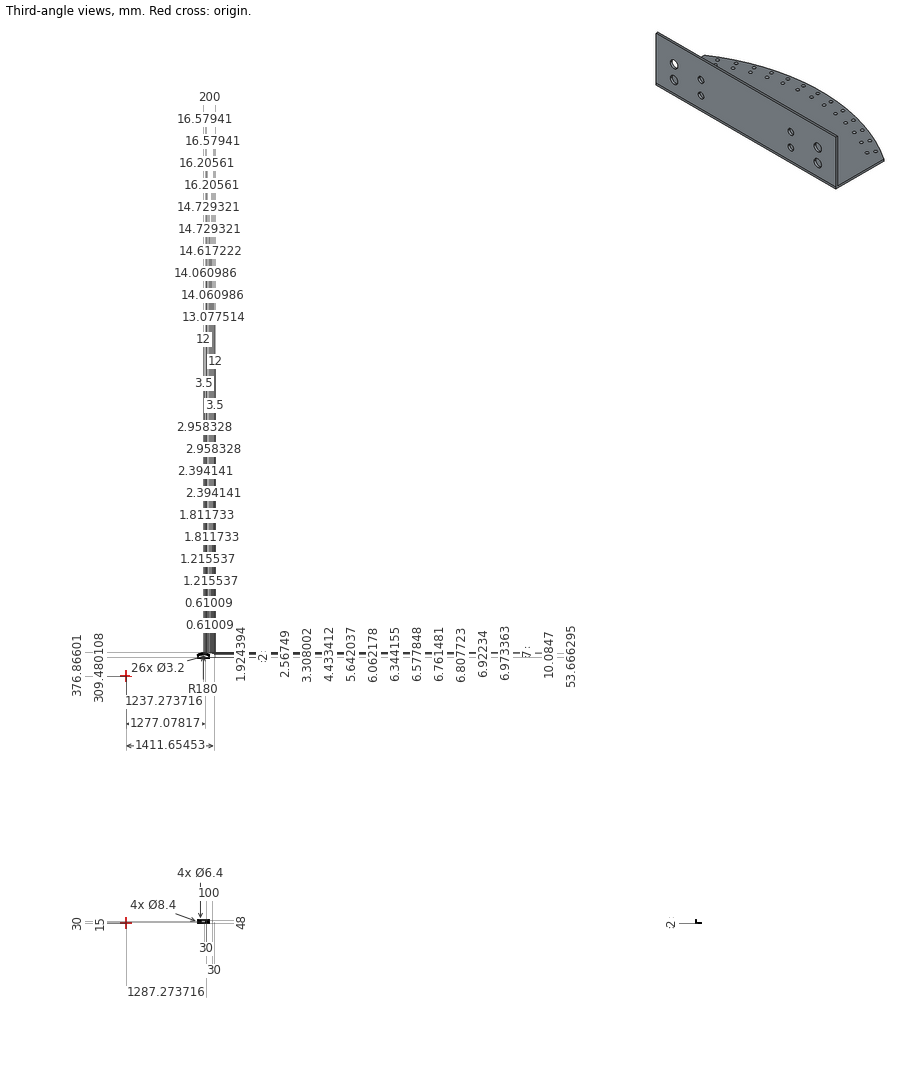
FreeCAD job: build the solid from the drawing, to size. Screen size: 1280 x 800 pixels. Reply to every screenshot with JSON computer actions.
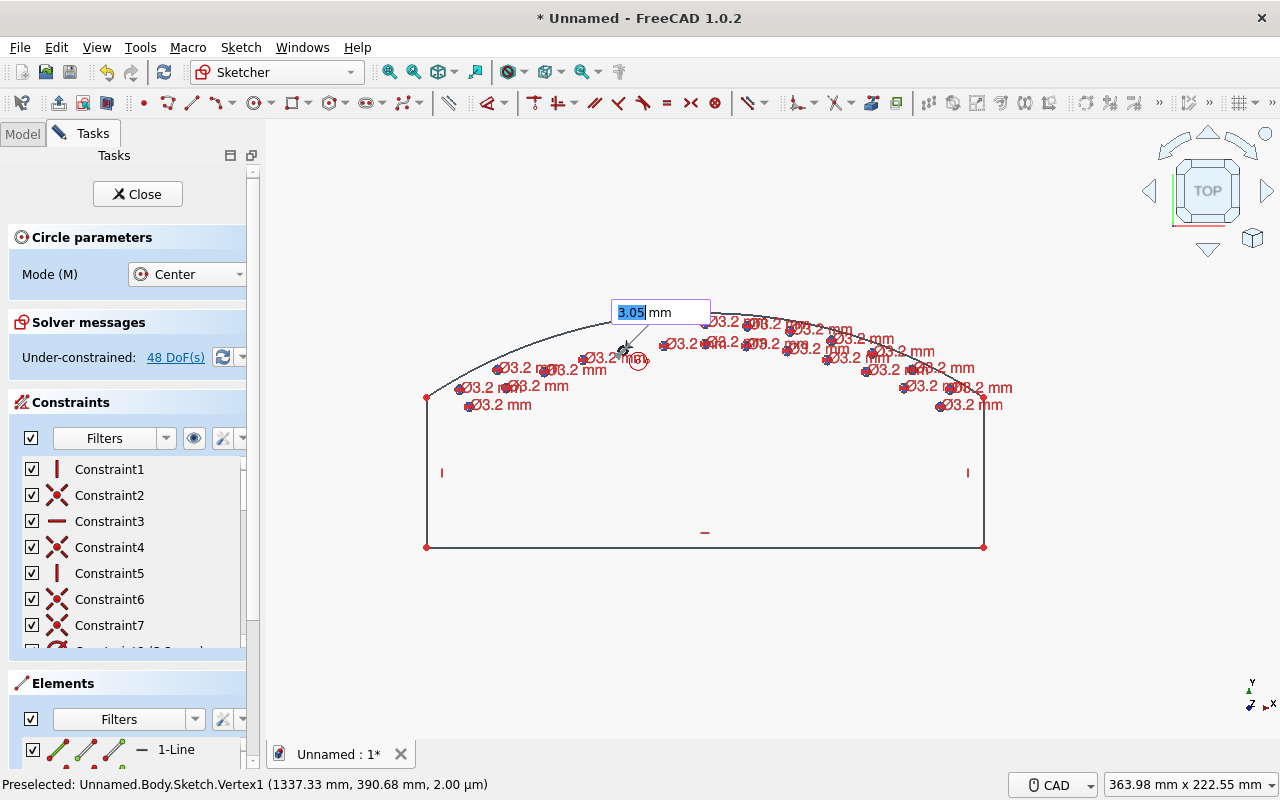
{"action": "type", "text": "3.2"}
{"action": "key", "text": "Return"}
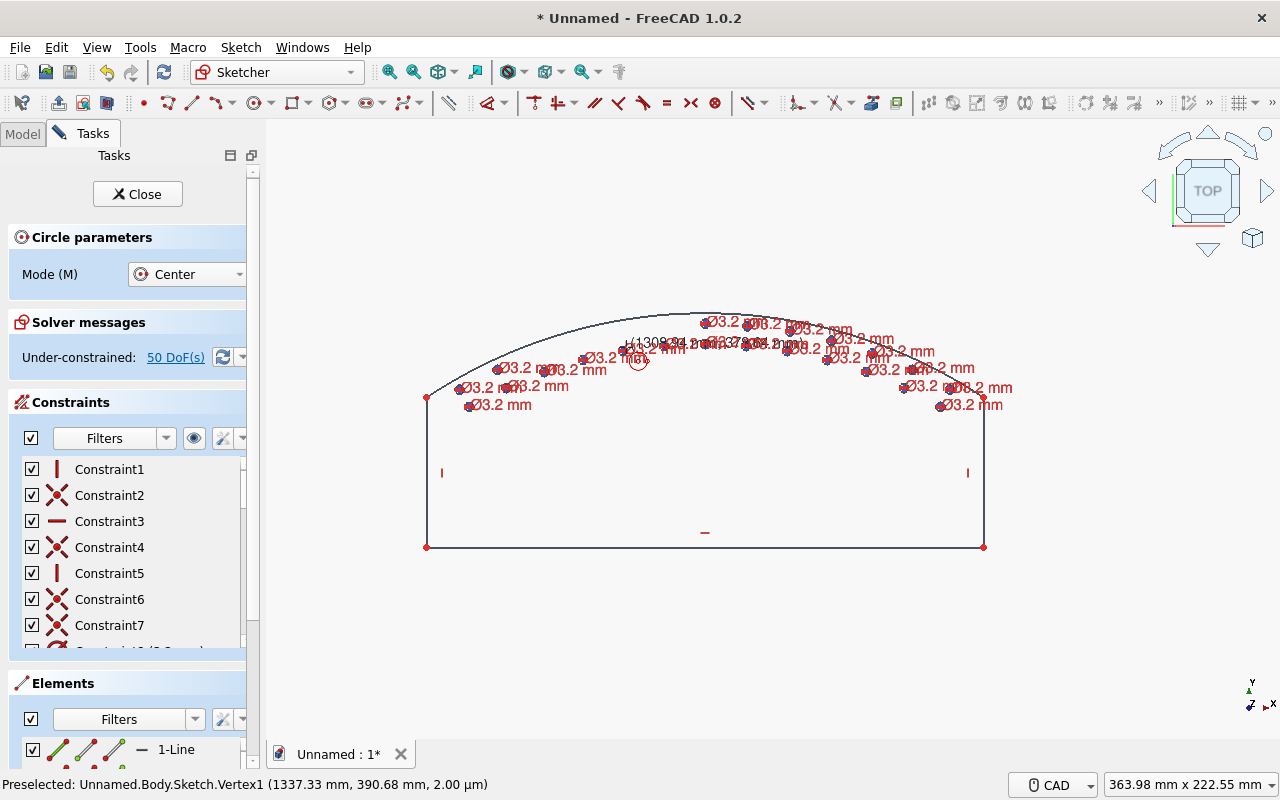
{"action": "scroll", "coordinate": [537, 353], "scroll_direction": "up", "scroll_amount": 9}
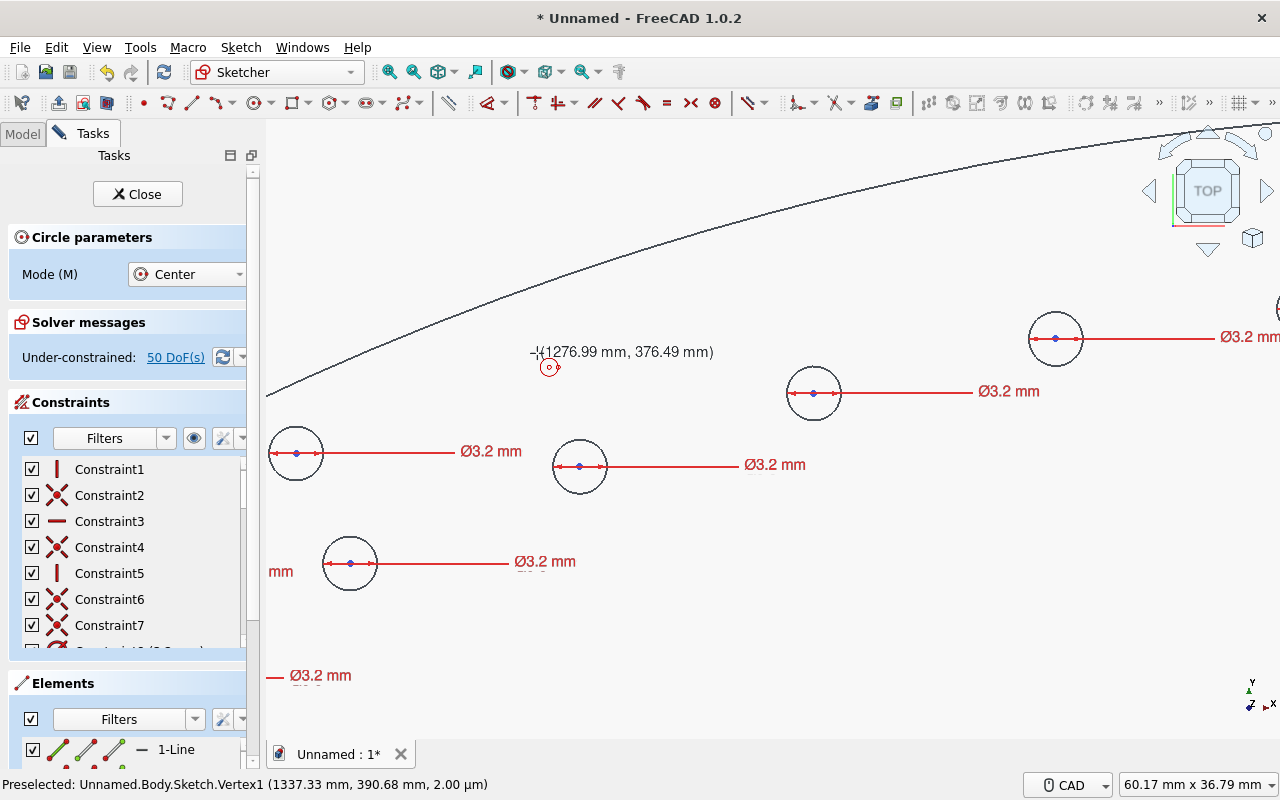
{"action": "scroll", "coordinate": [537, 353], "scroll_direction": "down", "scroll_amount": 9}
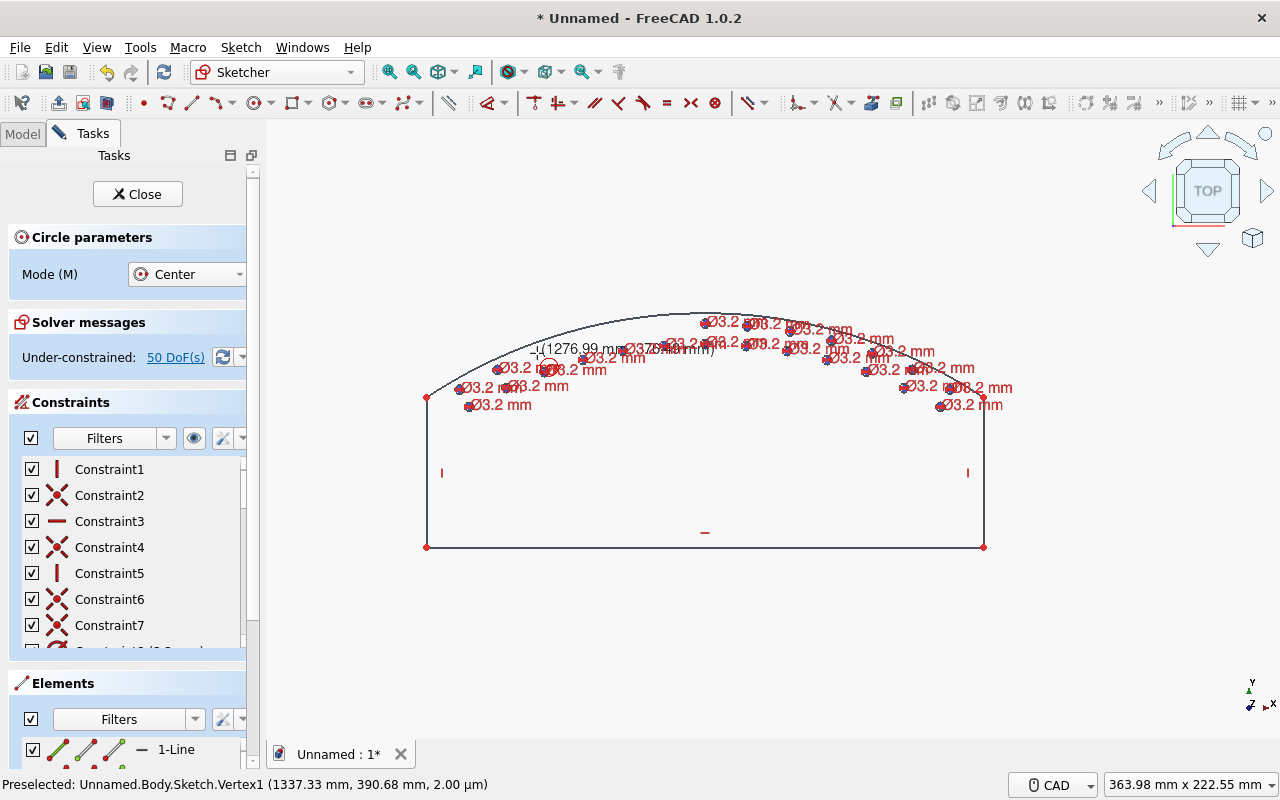
{"action": "scroll", "coordinate": [537, 353], "scroll_direction": "up", "scroll_amount": 2}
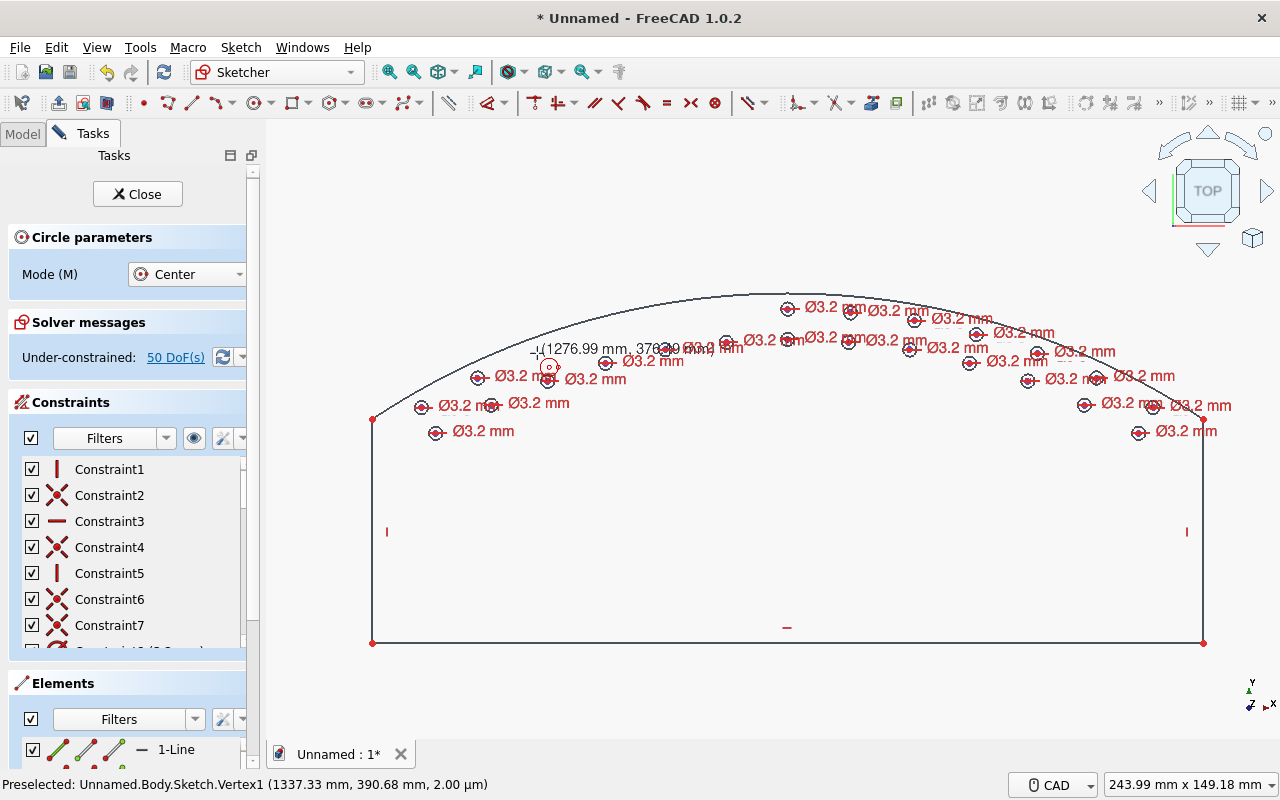
{"action": "left_click", "coordinate": [537, 353]}
{"action": "mouse_move", "coordinate": [542, 357]}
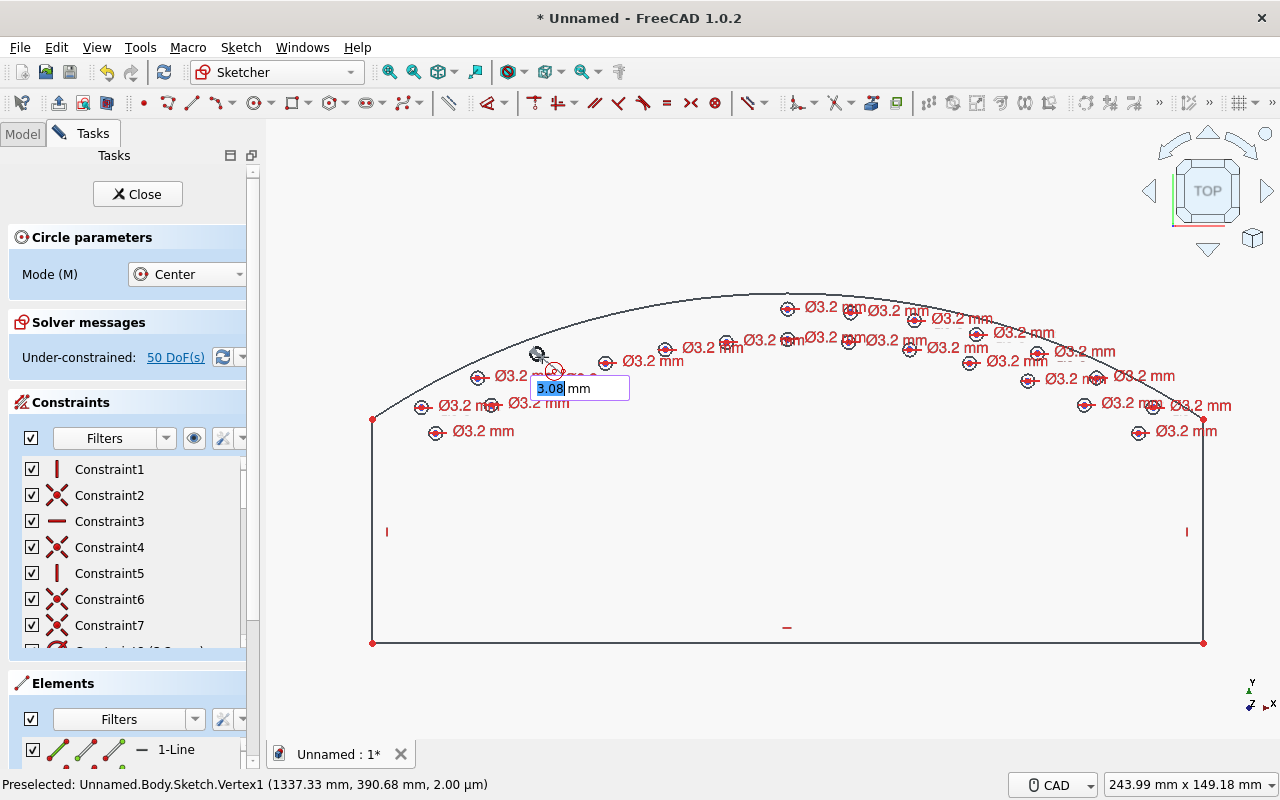
{"action": "type", "text": "3.2"}
{"action": "key", "text": "Return"}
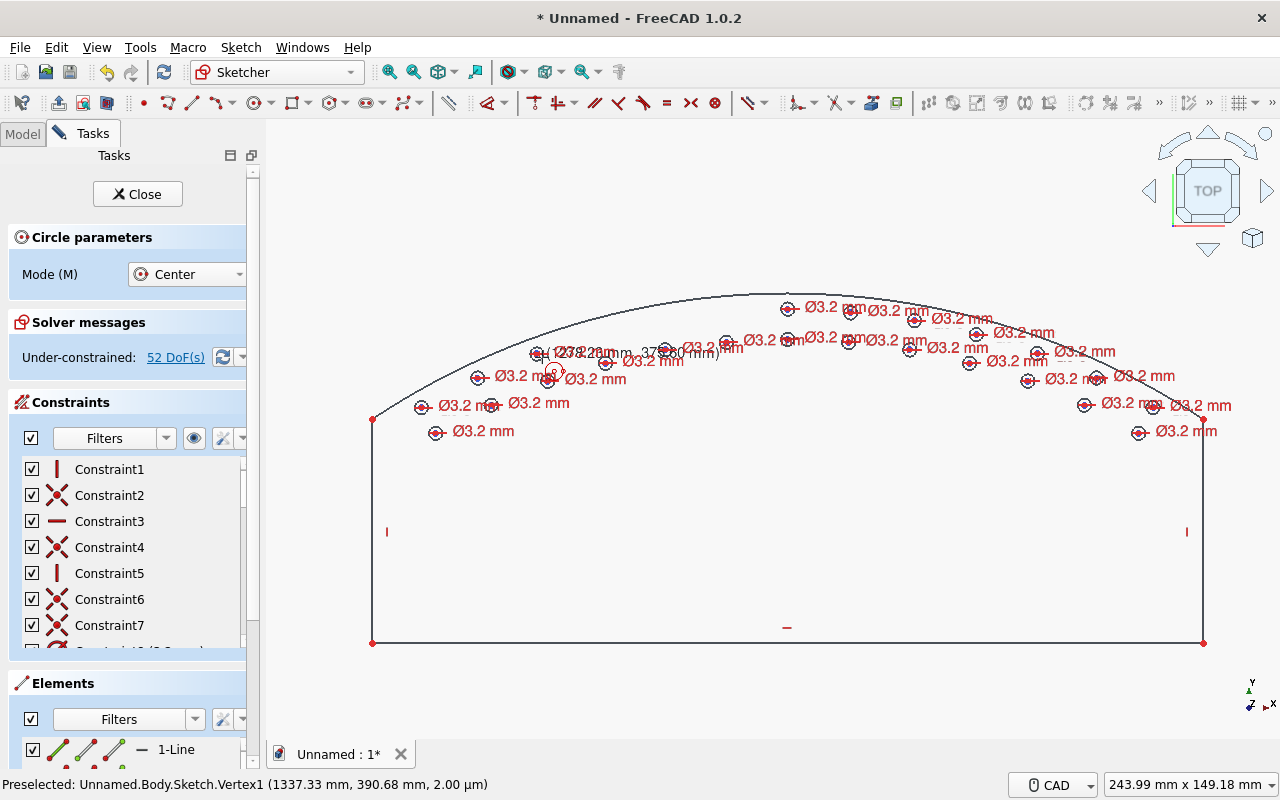
{"action": "scroll", "coordinate": [660, 320], "scroll_direction": "up", "scroll_amount": 7}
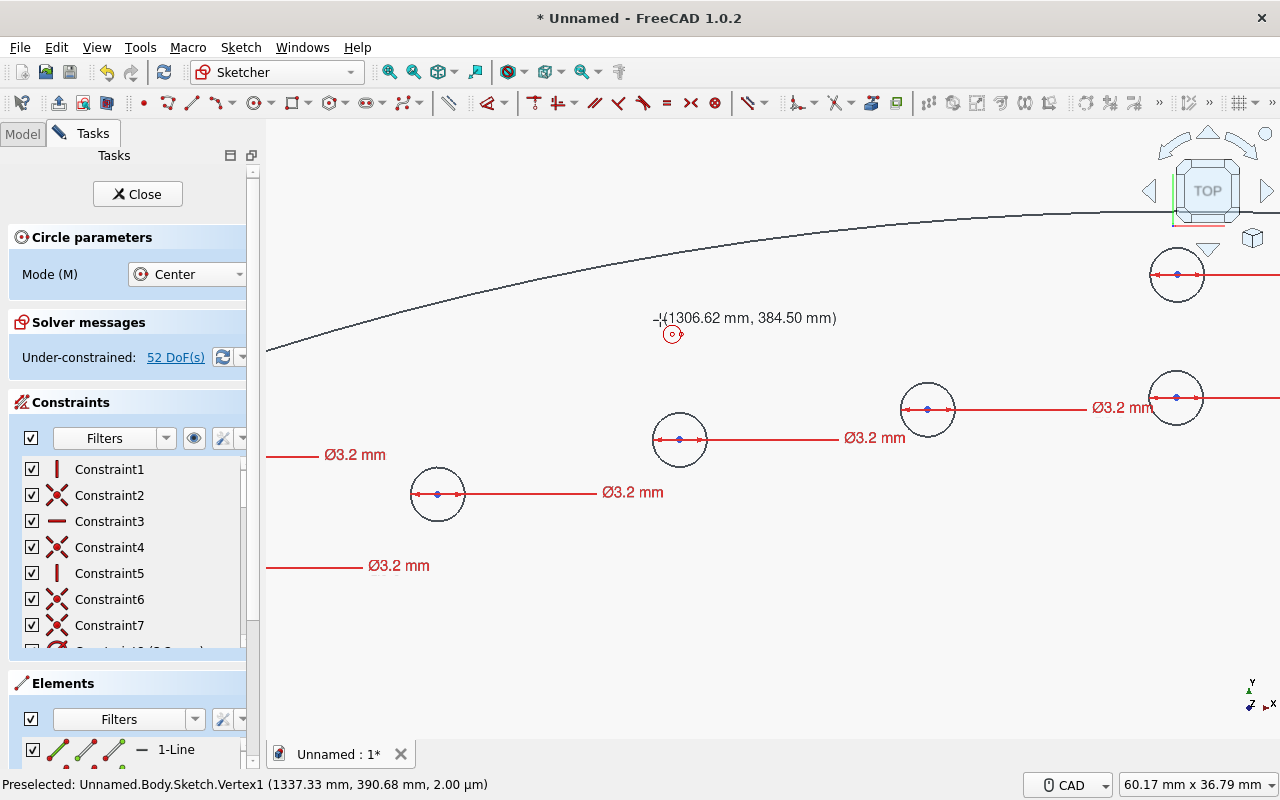
{"action": "scroll", "coordinate": [611, 333], "scroll_direction": "down", "scroll_amount": 9}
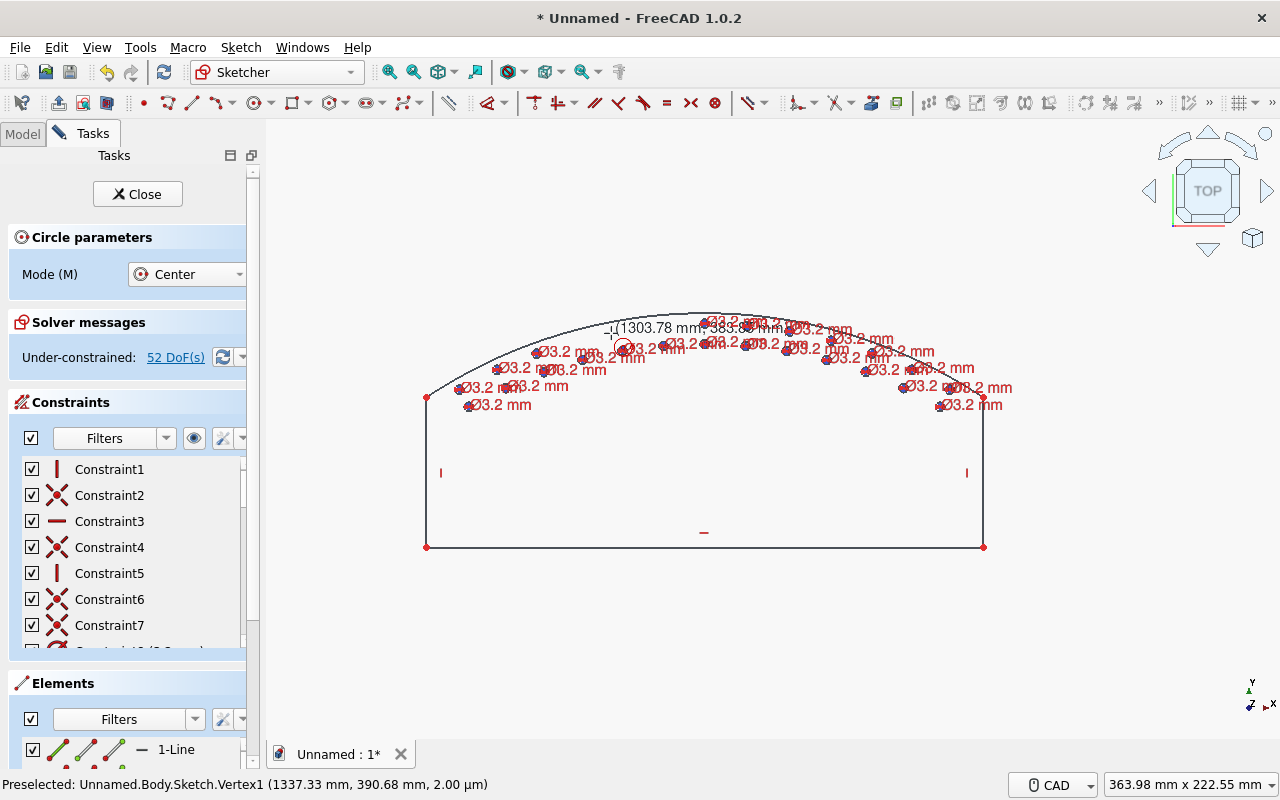
{"action": "scroll", "coordinate": [619, 331], "scroll_direction": "up", "scroll_amount": 2}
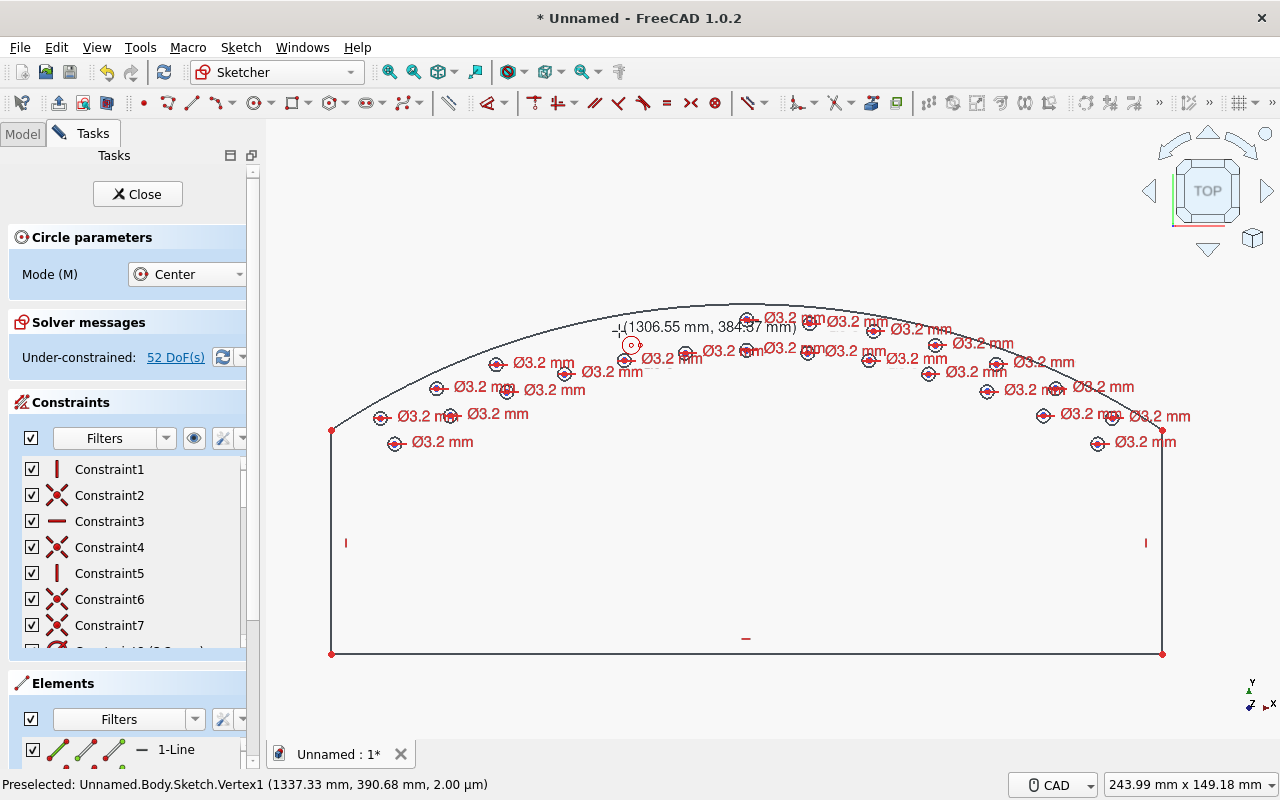
{"action": "left_click", "coordinate": [619, 331]}
{"action": "mouse_move", "coordinate": [624, 335]}